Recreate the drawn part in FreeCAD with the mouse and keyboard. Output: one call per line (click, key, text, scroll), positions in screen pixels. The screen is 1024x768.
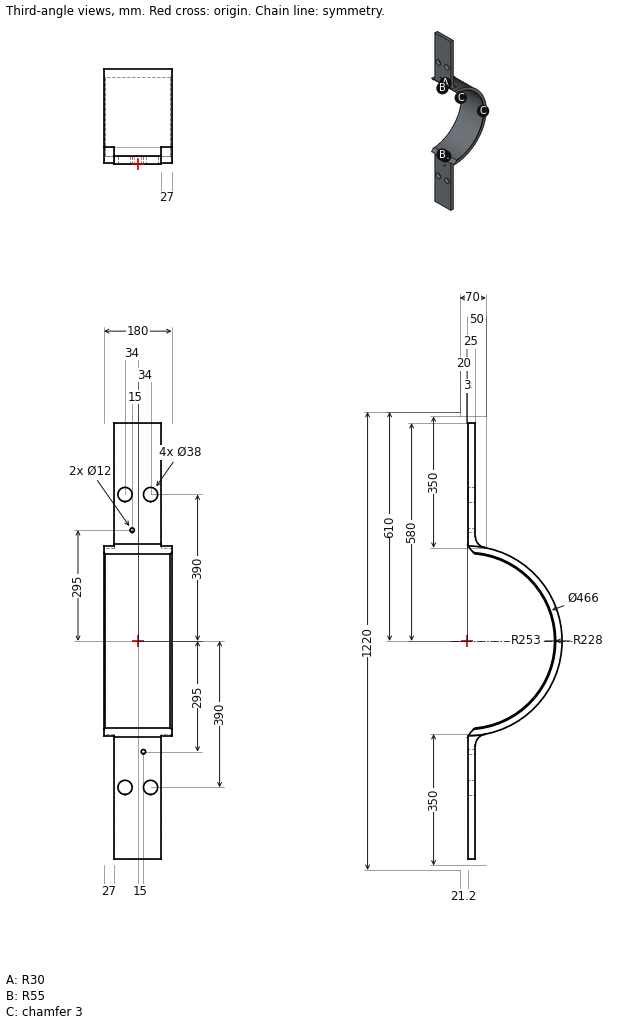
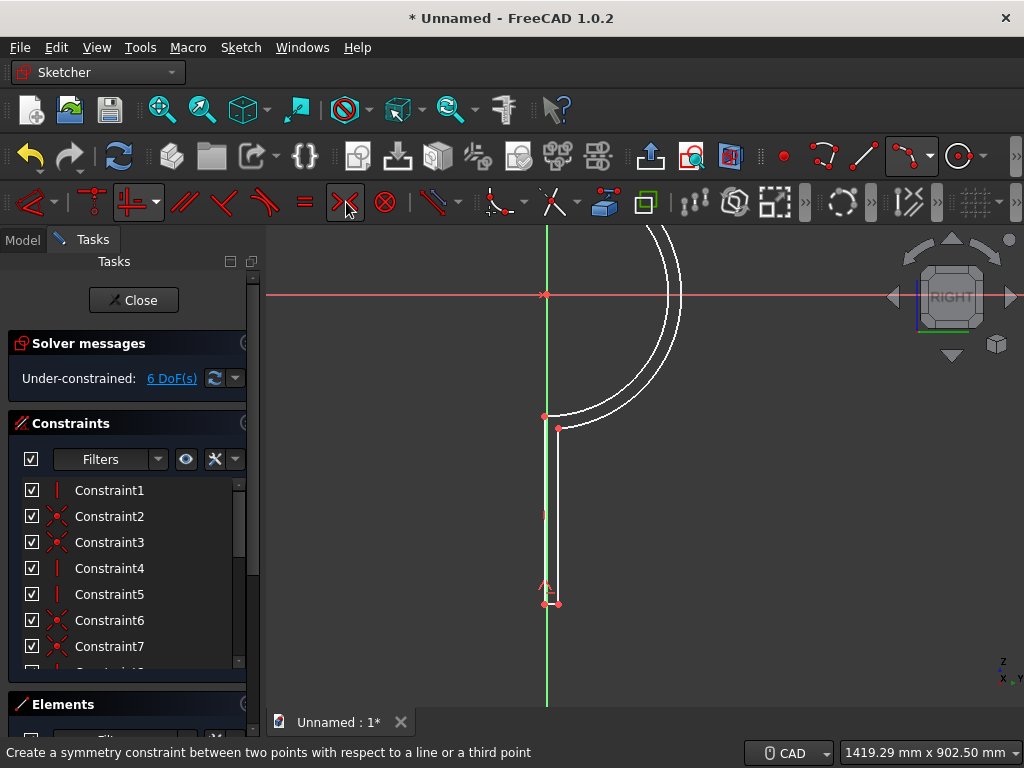
click(30, 202)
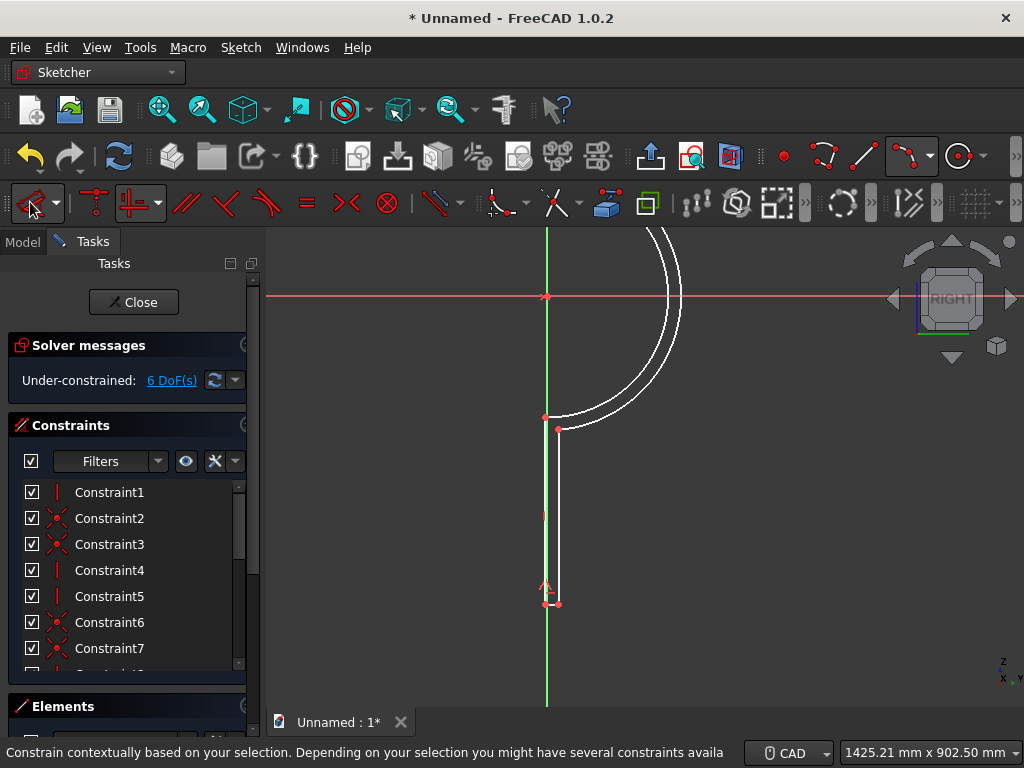
click(645, 368)
click(671, 387)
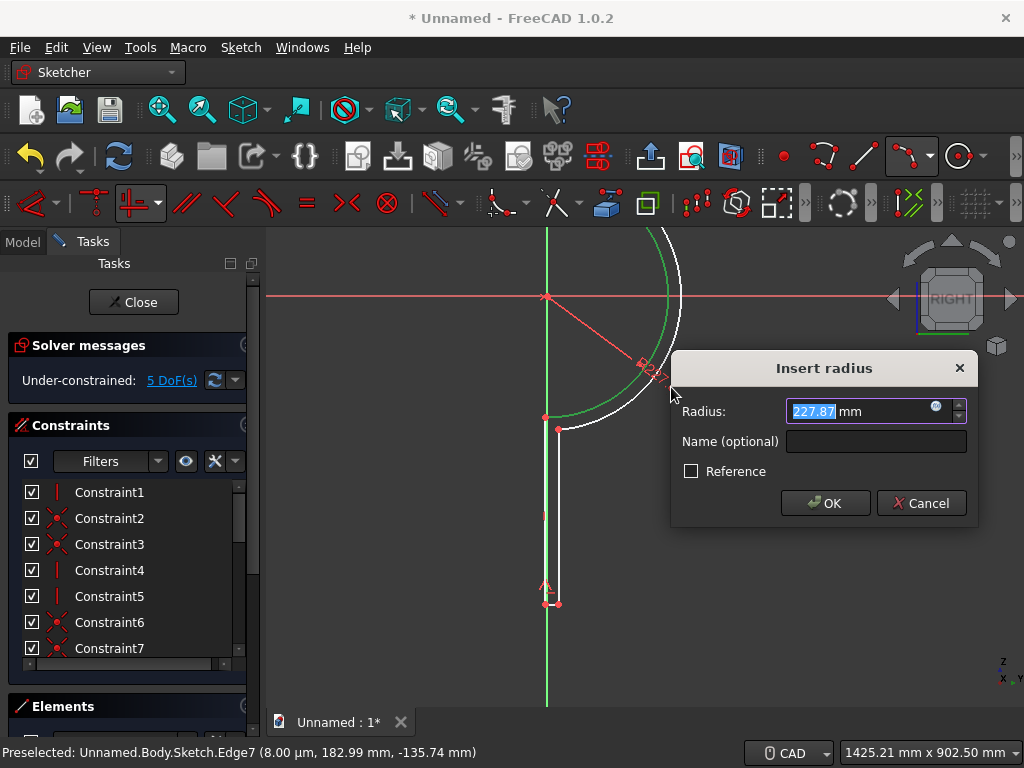
text(228)
key(Return)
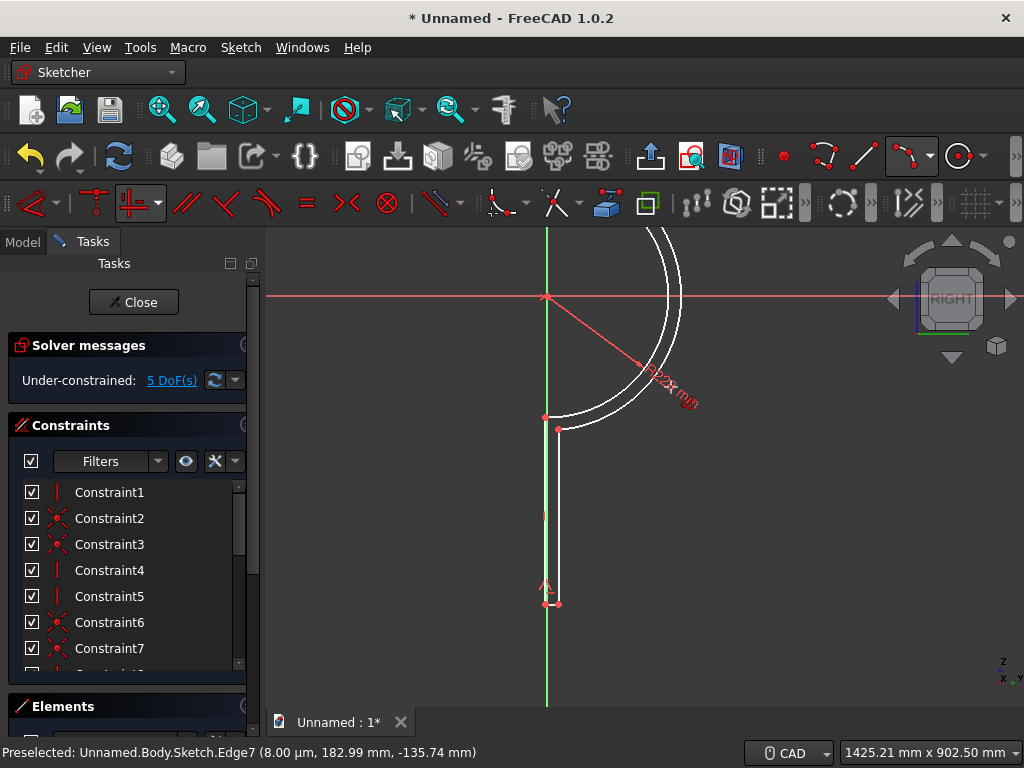
click(658, 371)
click(623, 443)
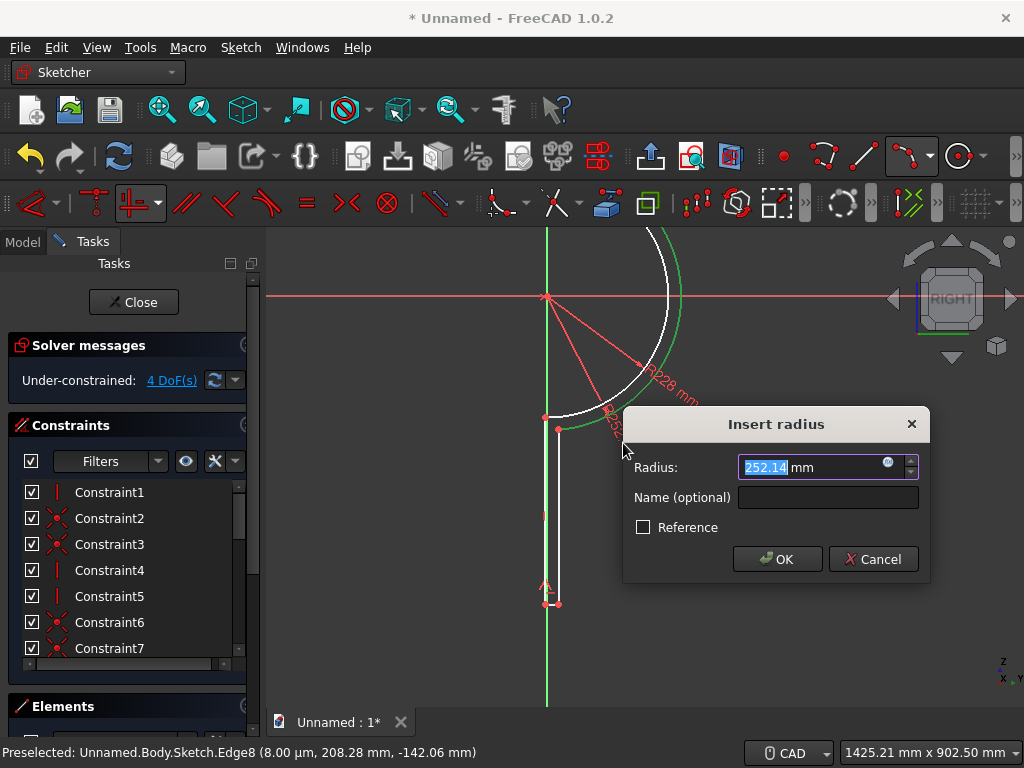
text(253)
key(Return)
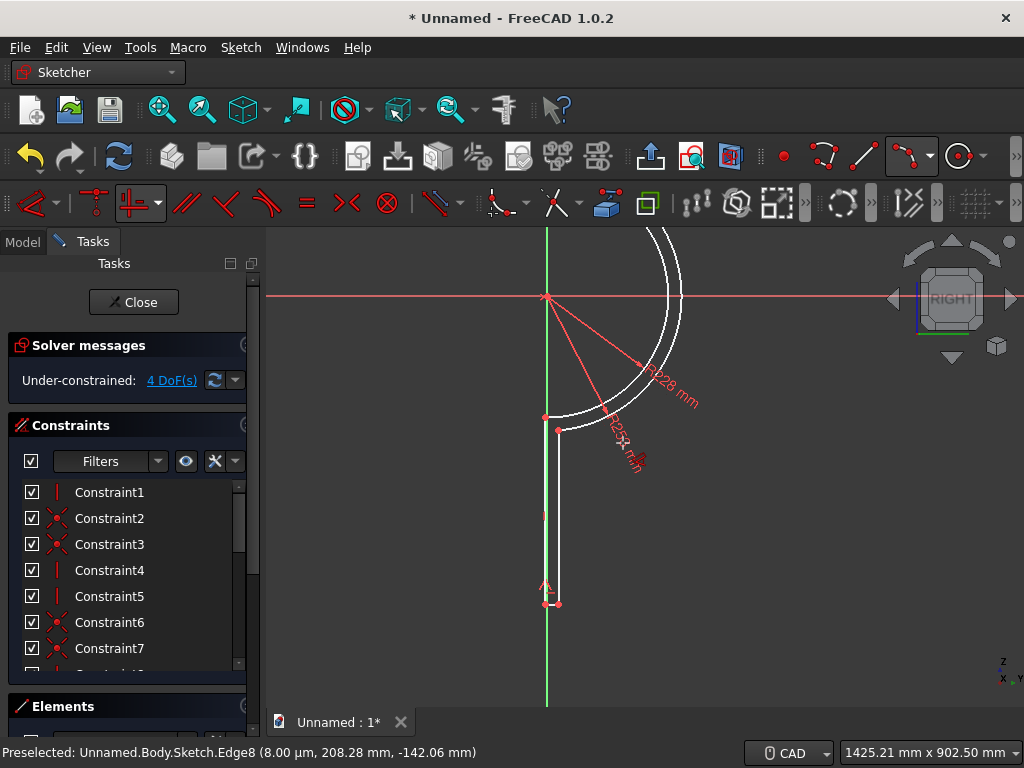
scroll(546, 606, down, 4)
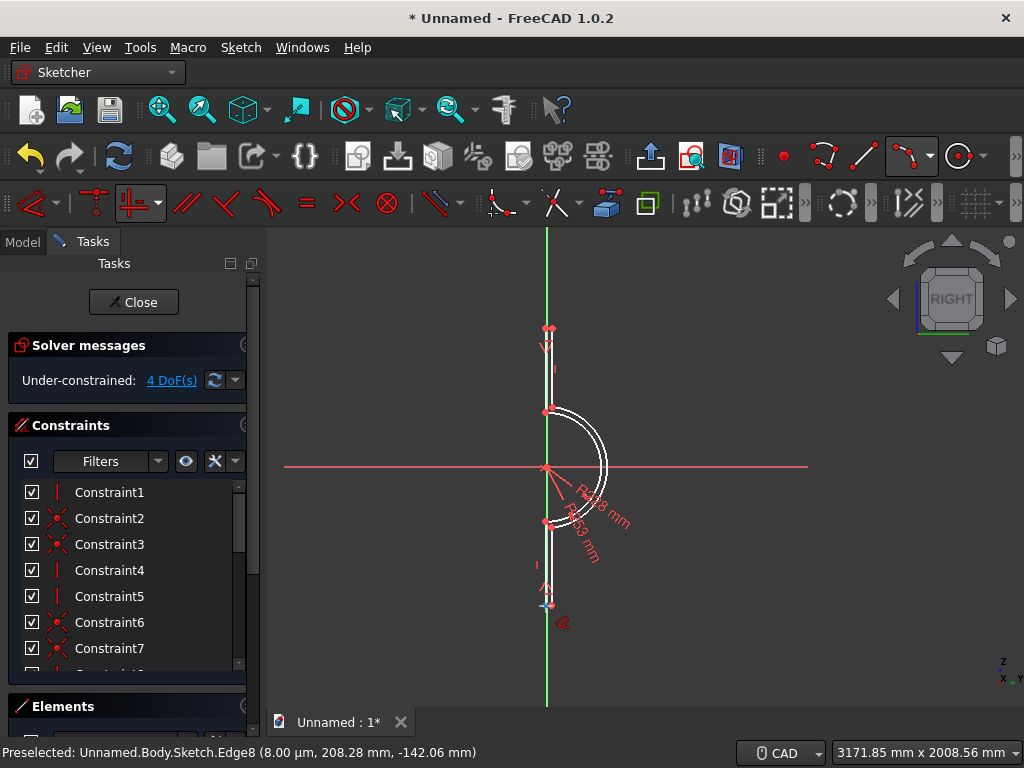
scroll(550, 329, up, 10)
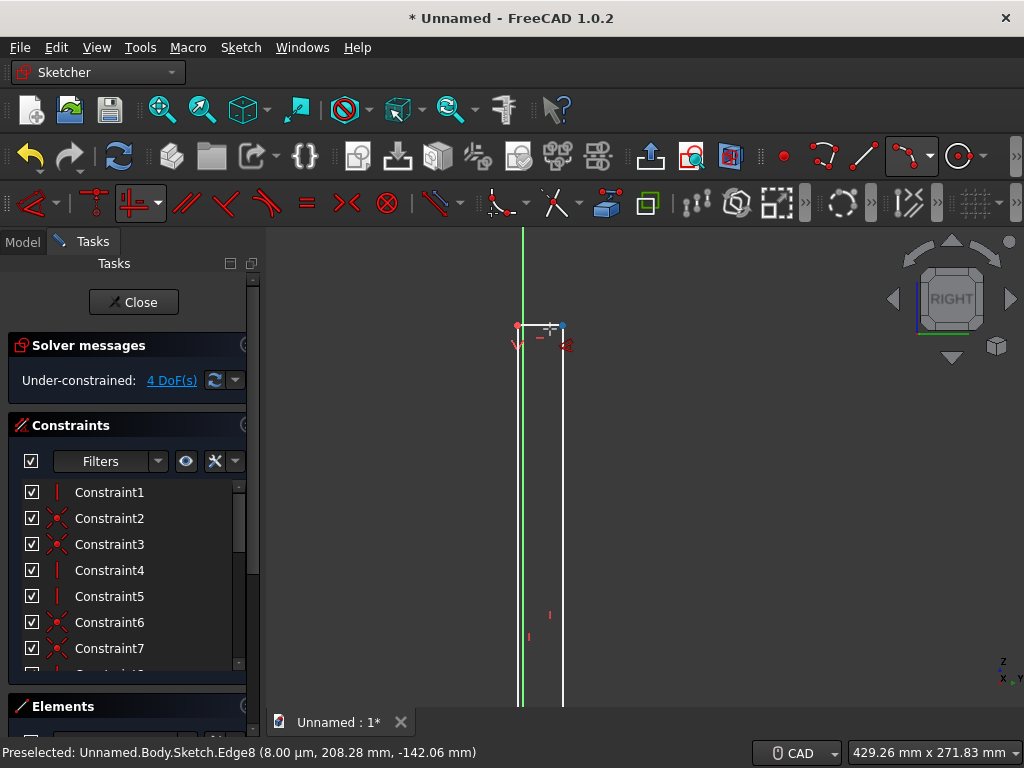
click(545, 325)
click(540, 291)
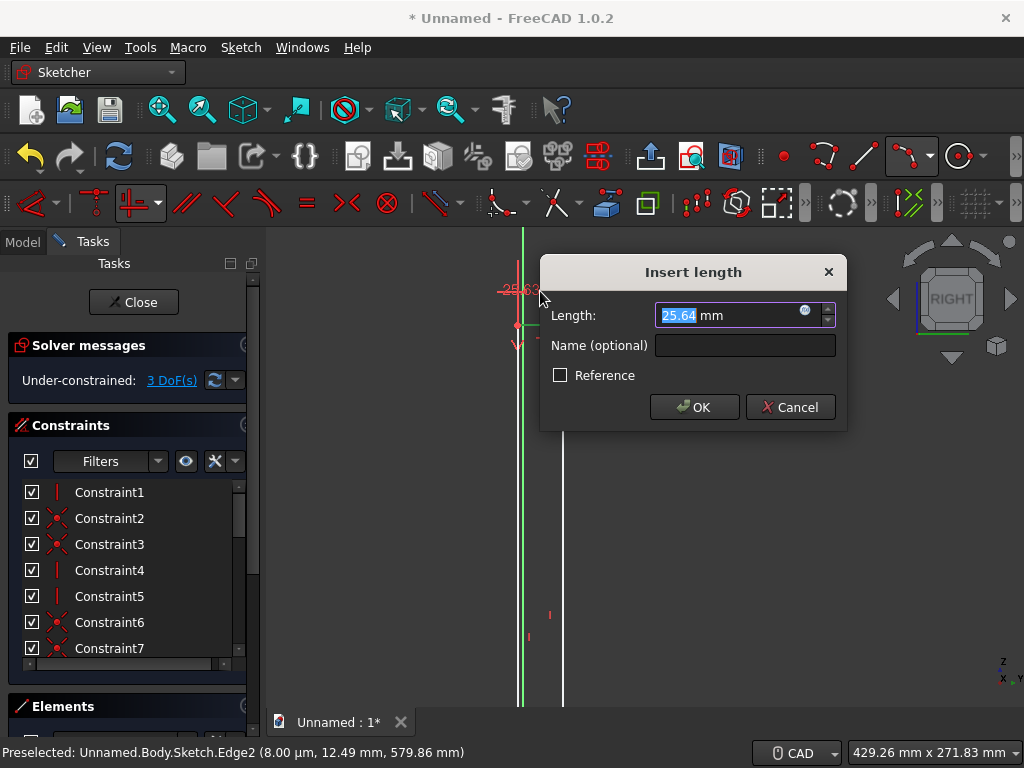
text(25)
key(Return)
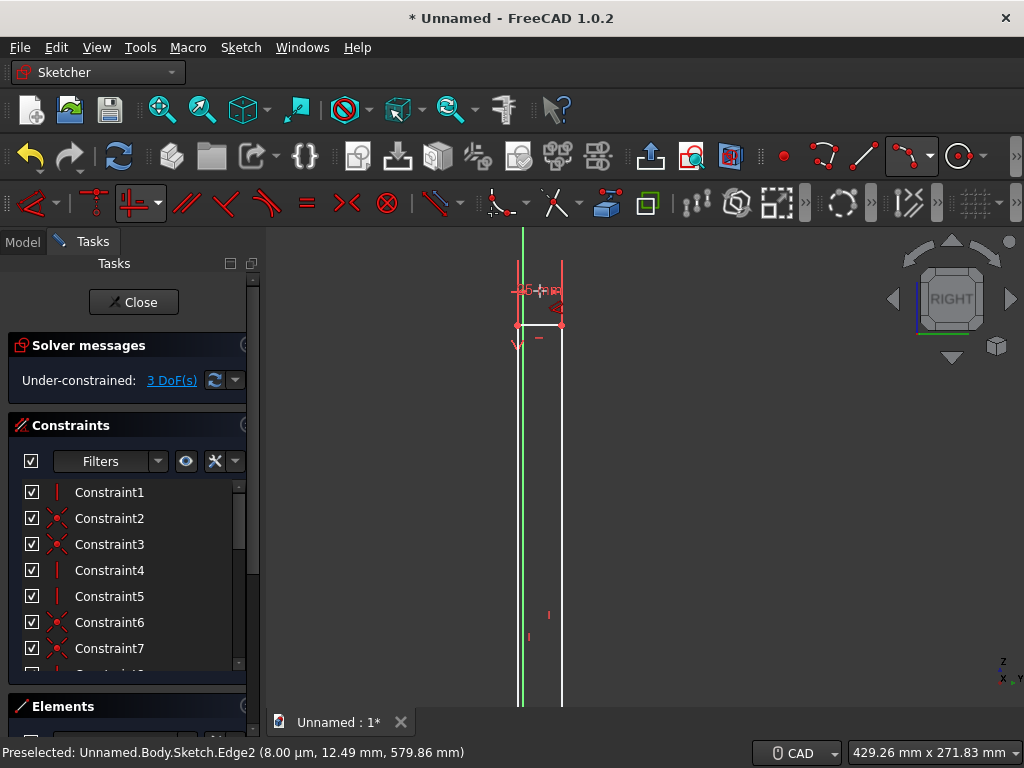
scroll(550, 329, down, 10)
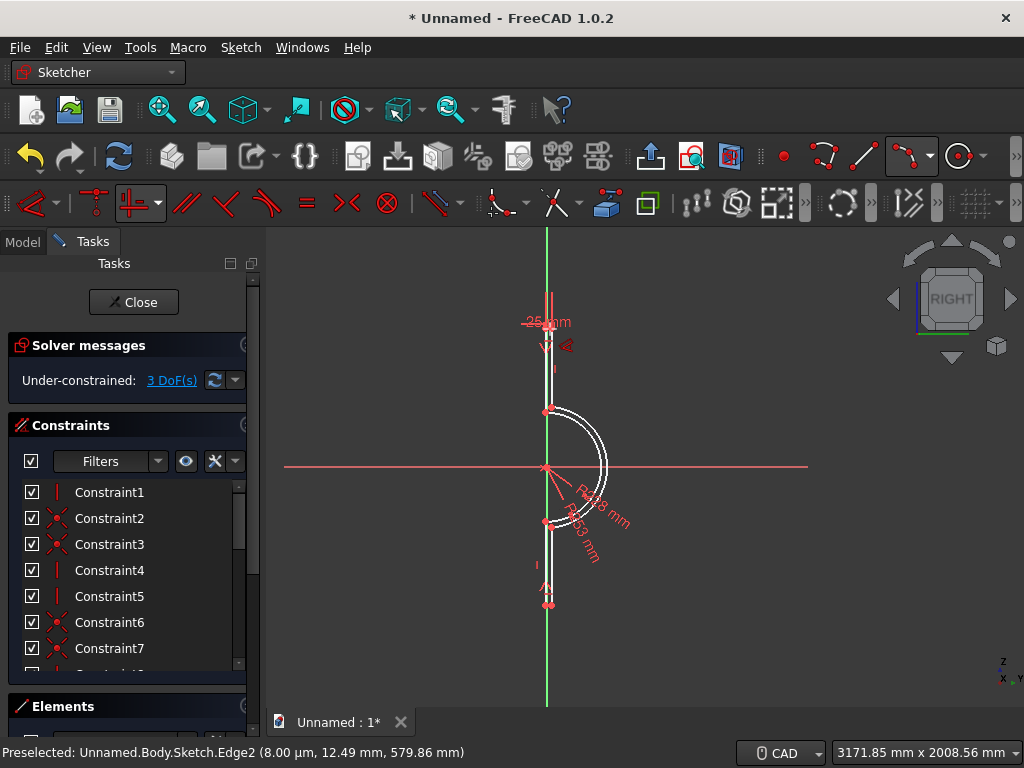
scroll(550, 606, up, 11)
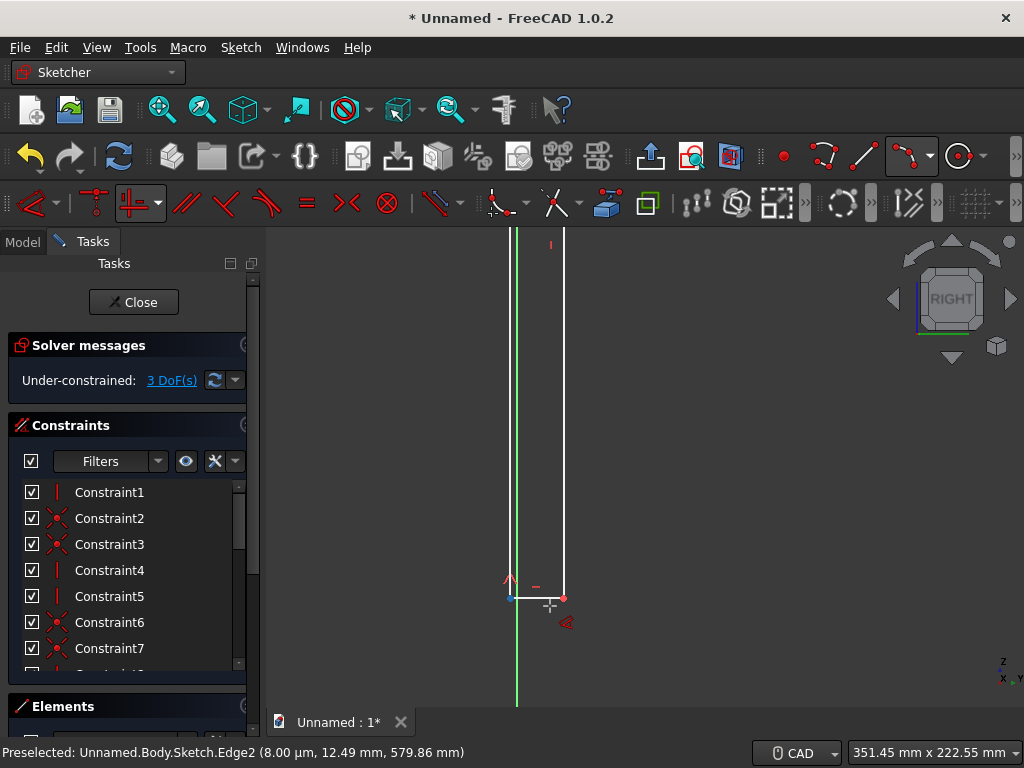
click(548, 598)
click(537, 632)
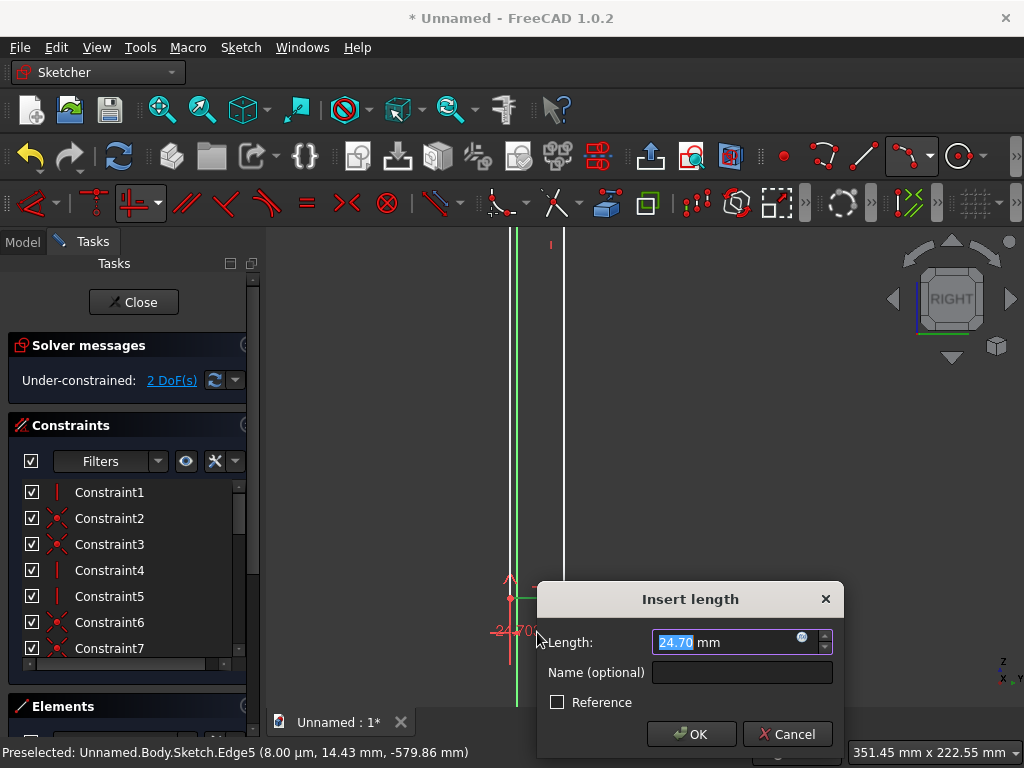
text(25)
key(Return)